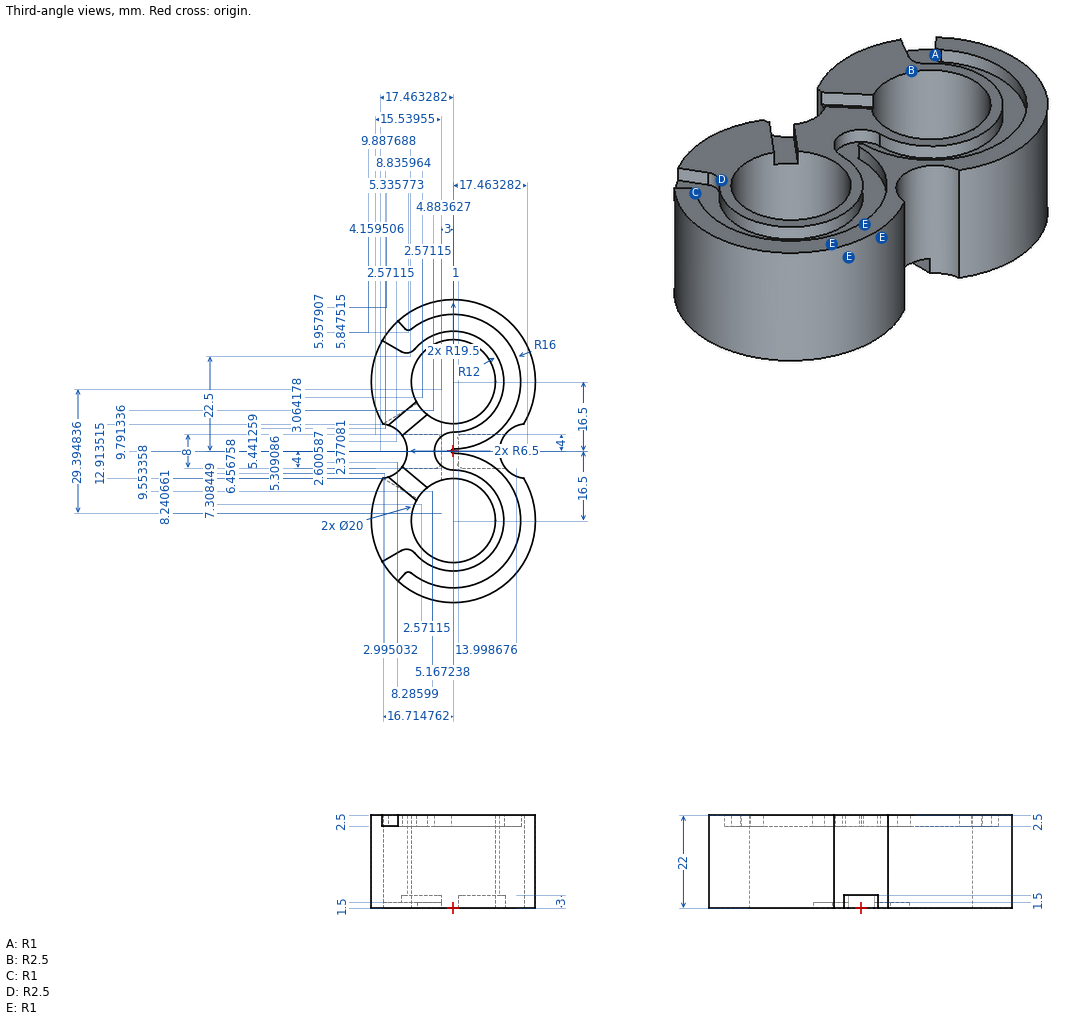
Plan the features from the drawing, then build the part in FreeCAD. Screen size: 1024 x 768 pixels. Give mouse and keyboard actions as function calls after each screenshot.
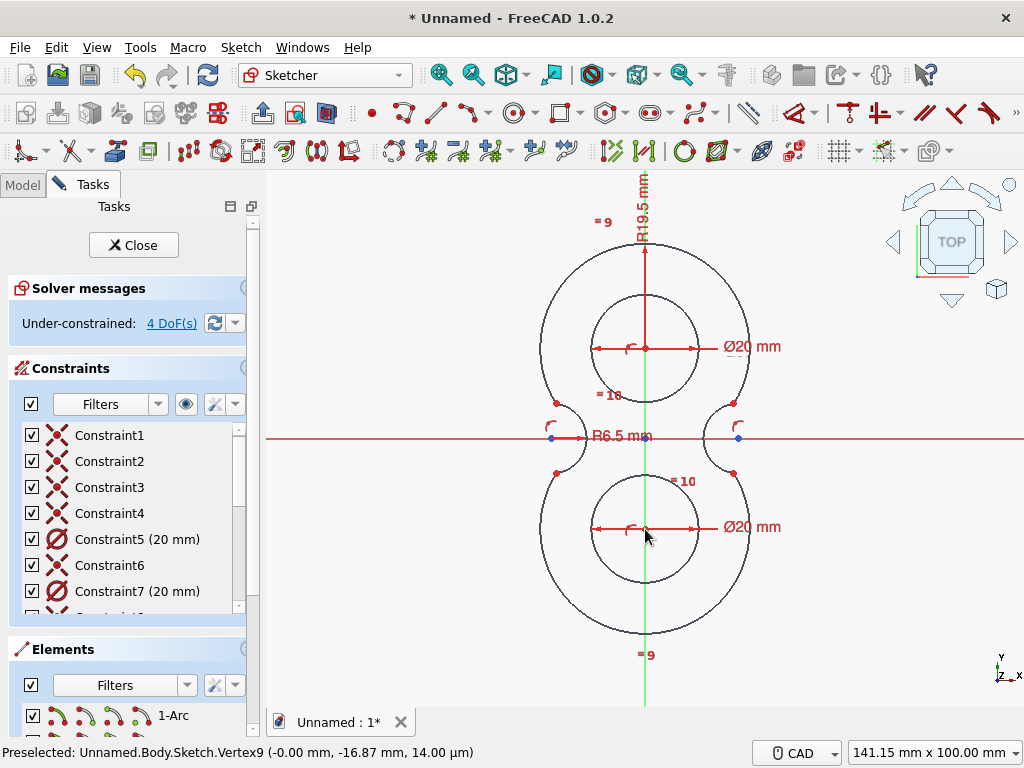
key(i)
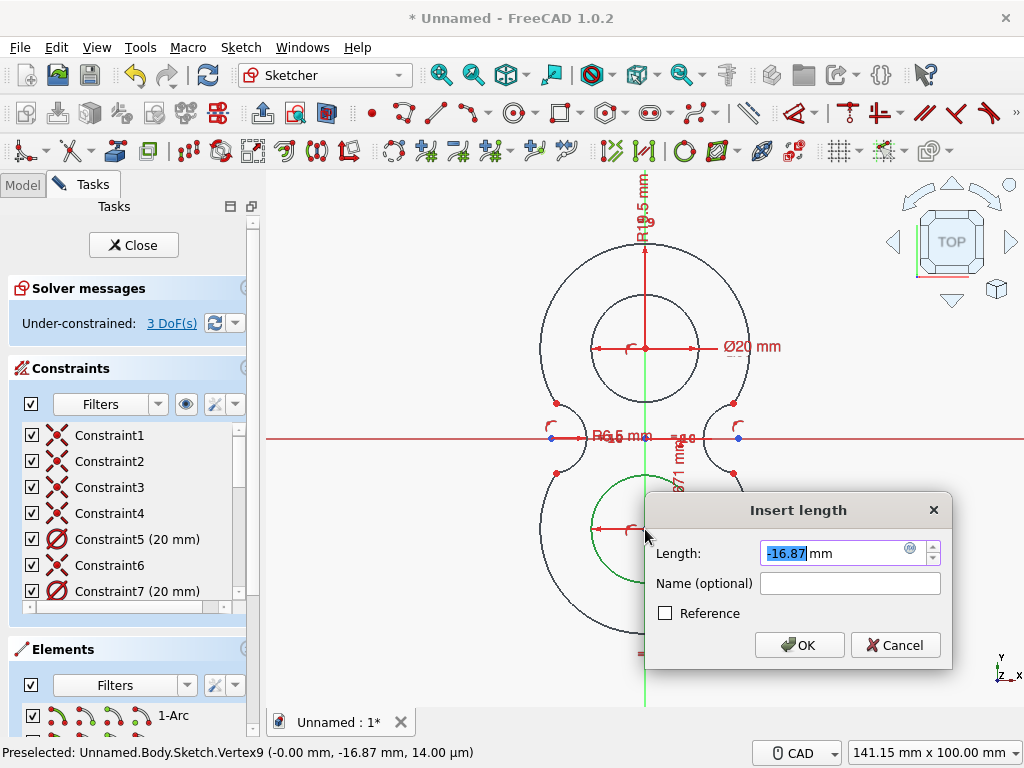
text(-16.5)
key(Return)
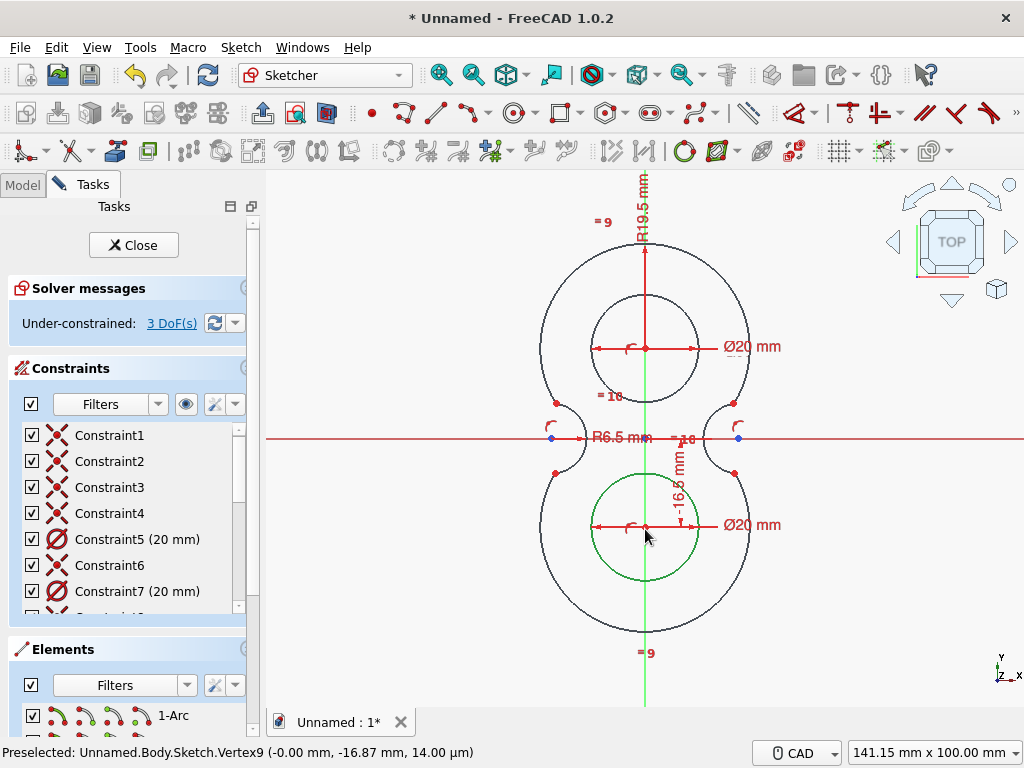
click(645, 349)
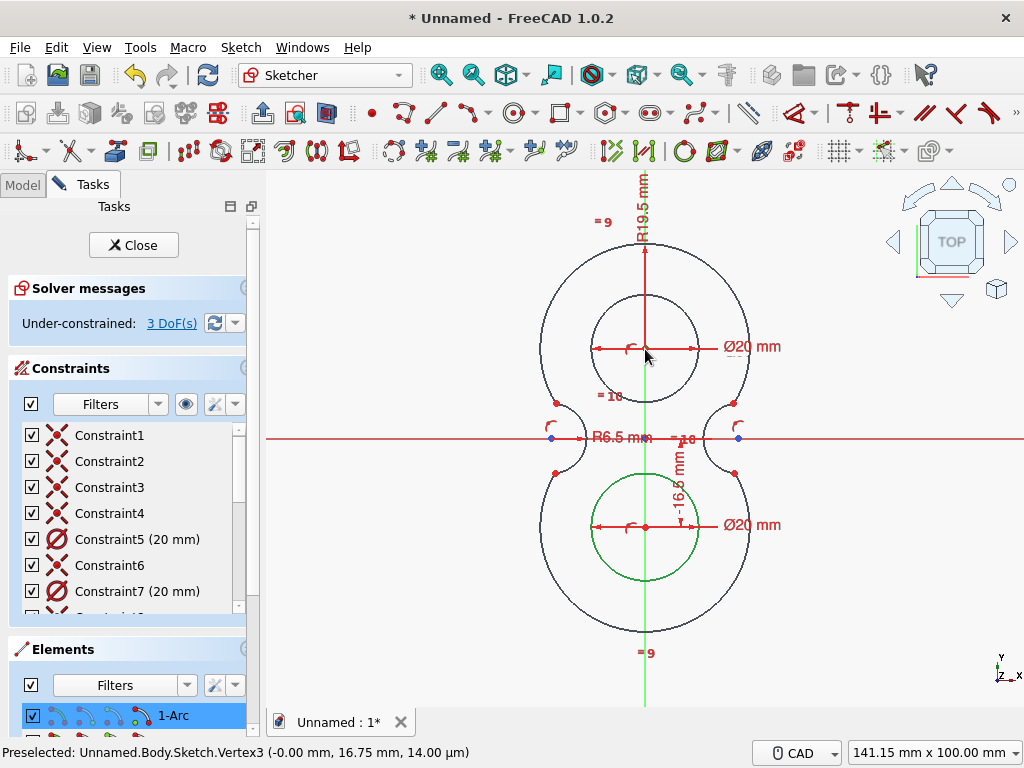
key(i)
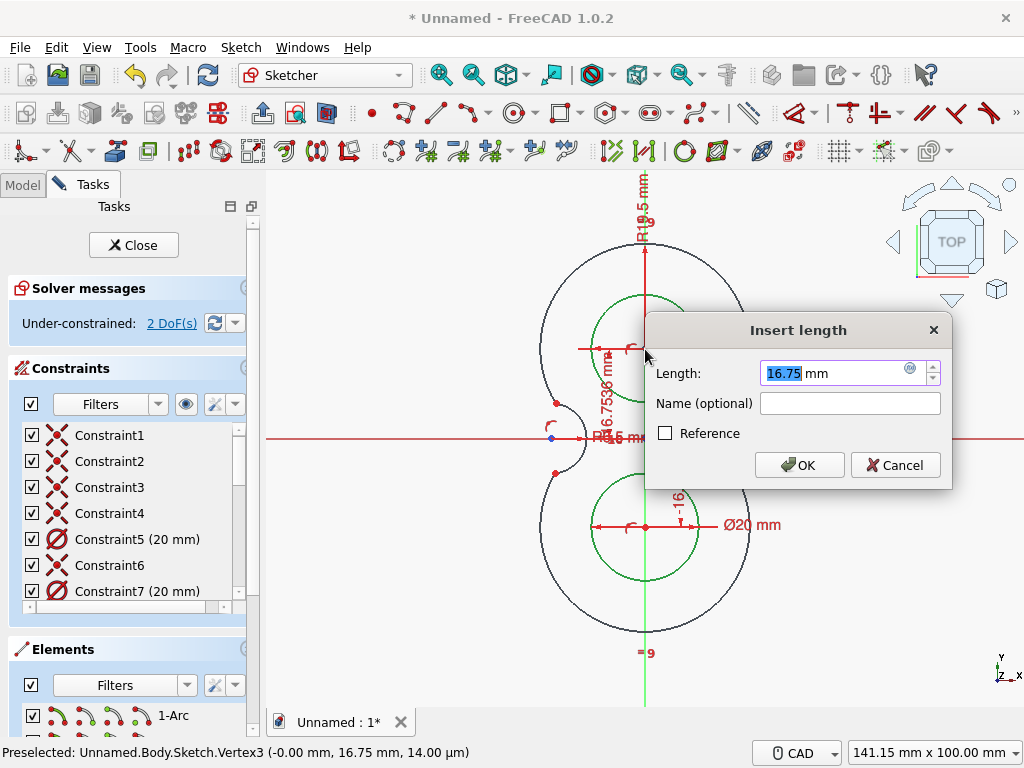
text(16.5)
key(Return)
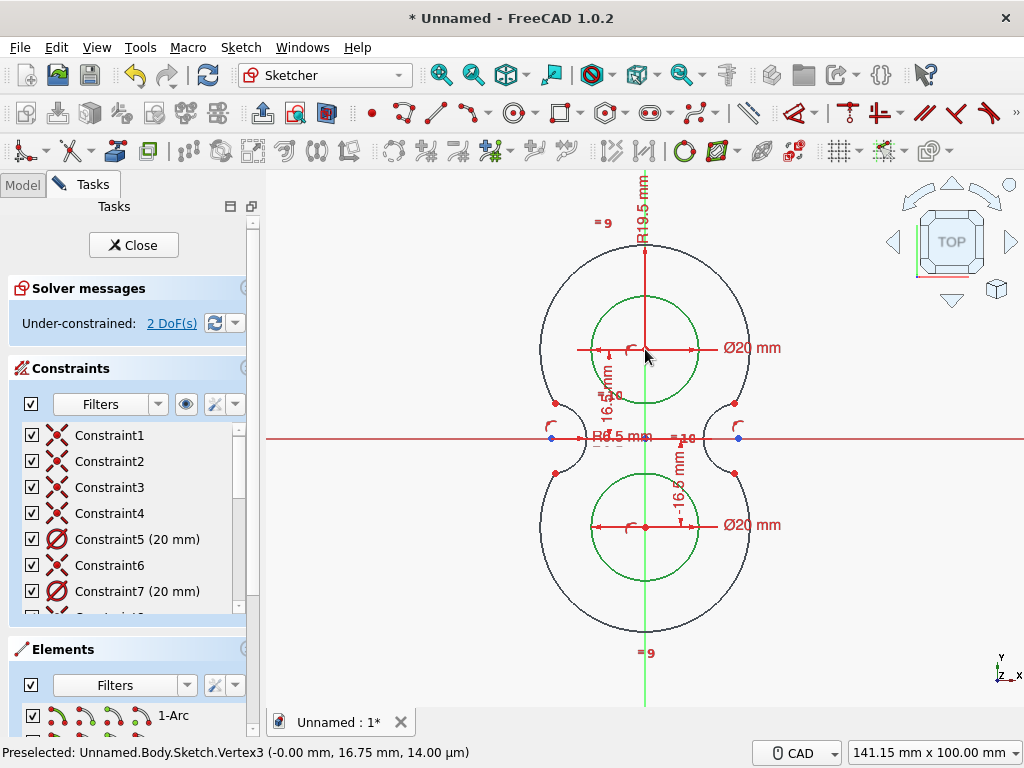
click(552, 438)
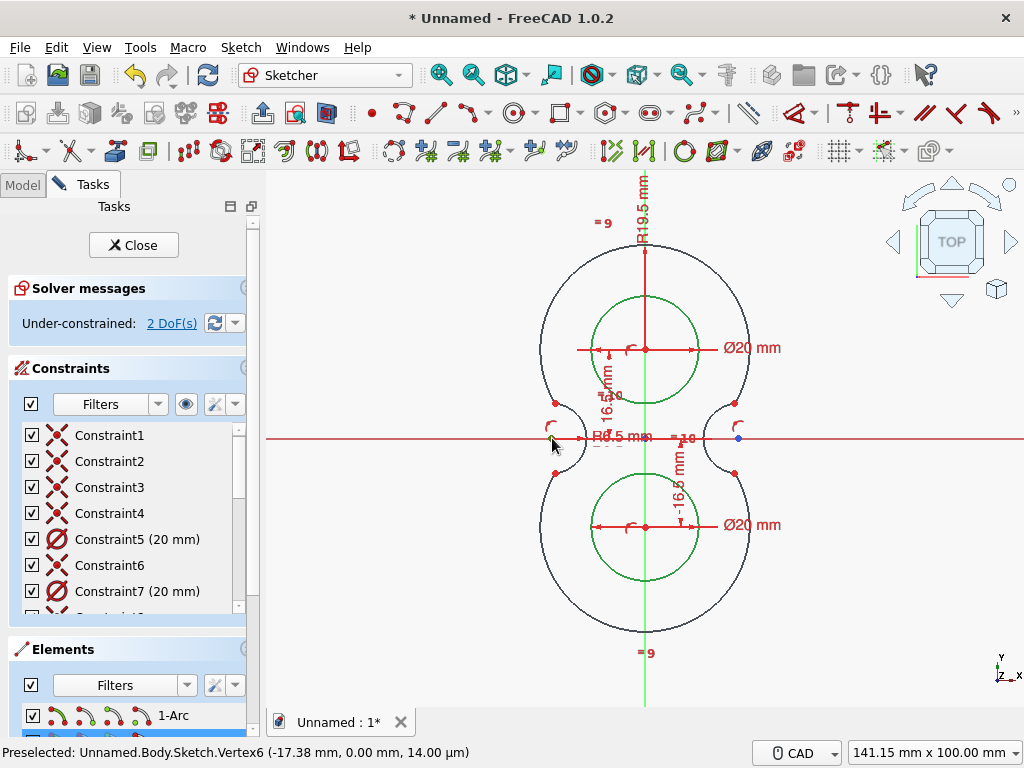
key(l)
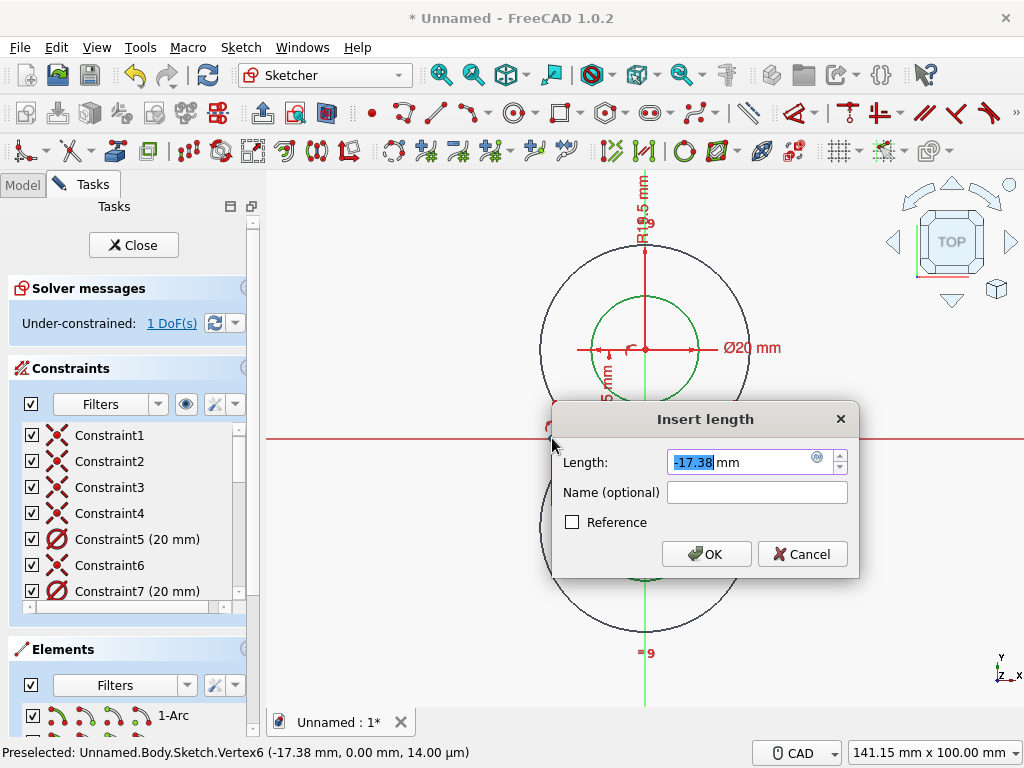
text(-17.463282)
key(Return)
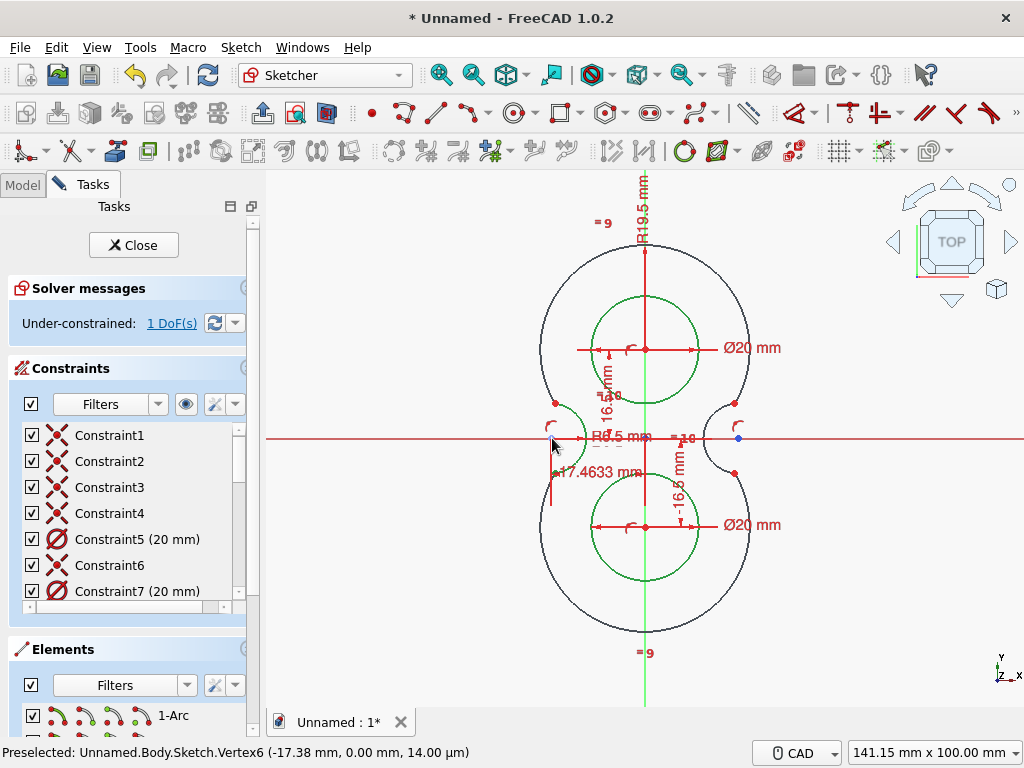
click(738, 438)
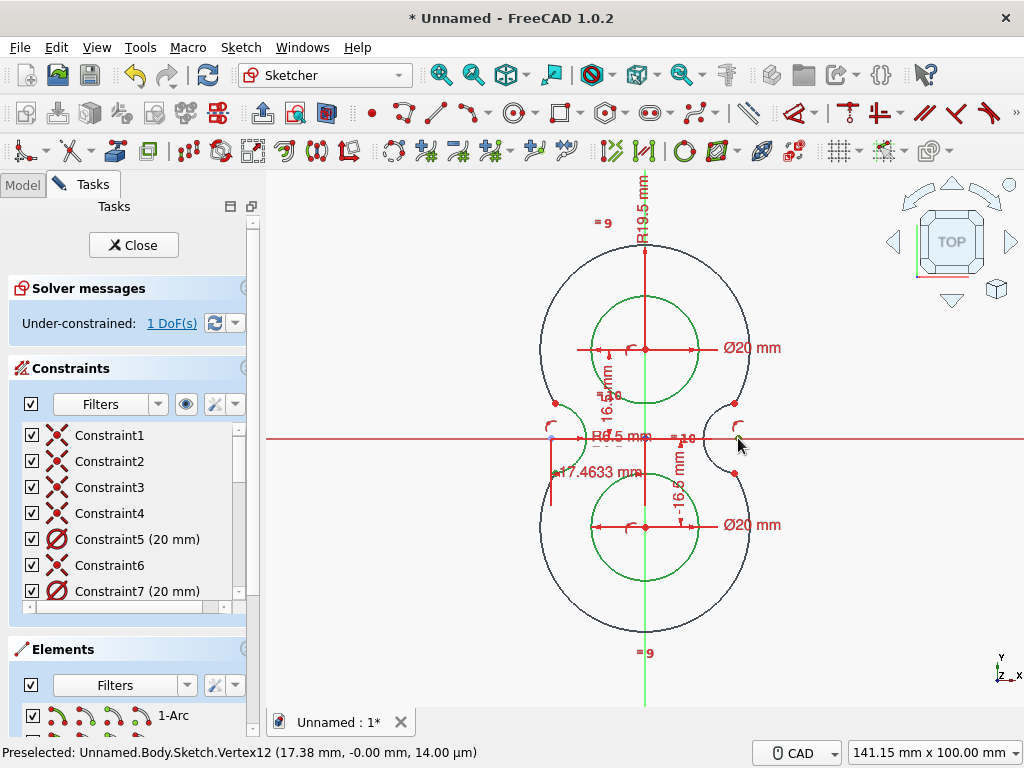
key(l)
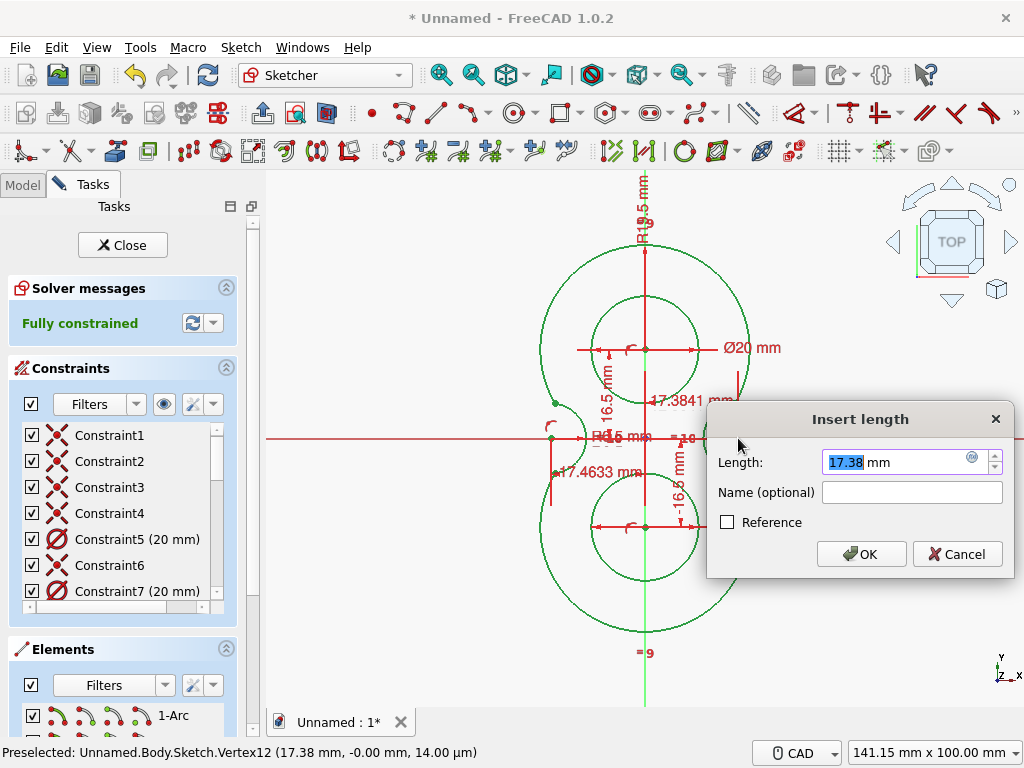
text(17.463282)
key(Return)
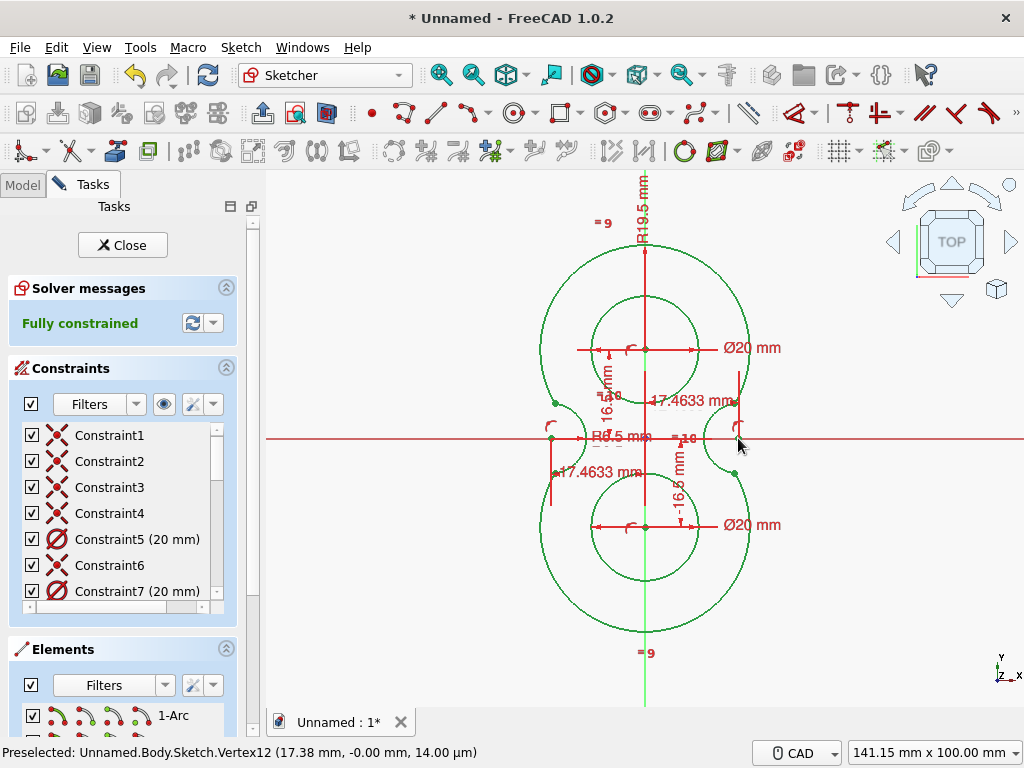
click(123, 245)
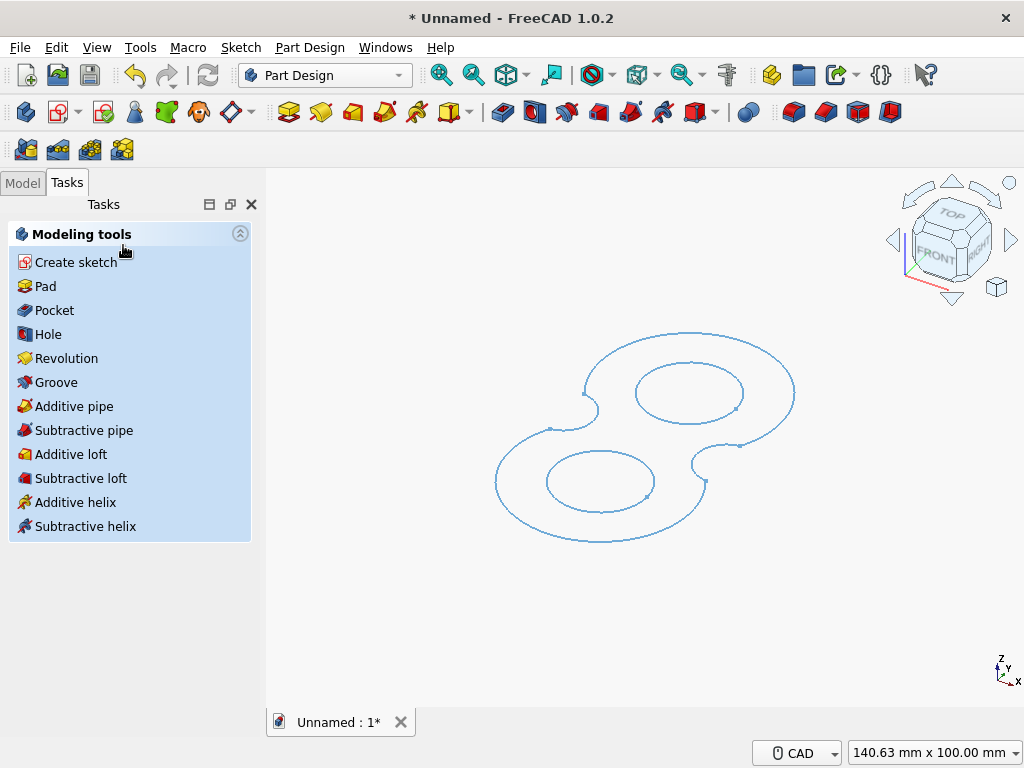
click(290, 112)